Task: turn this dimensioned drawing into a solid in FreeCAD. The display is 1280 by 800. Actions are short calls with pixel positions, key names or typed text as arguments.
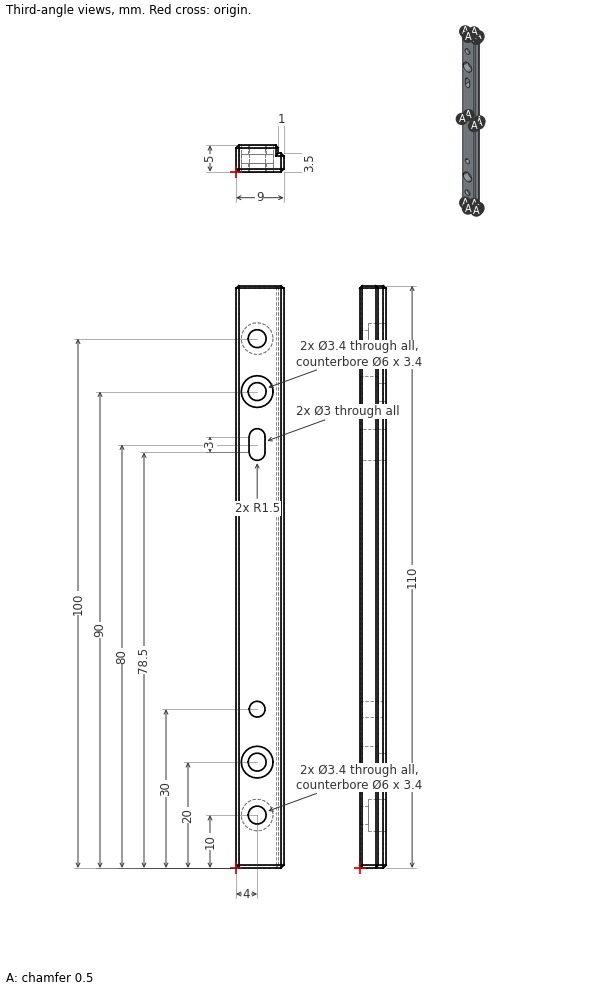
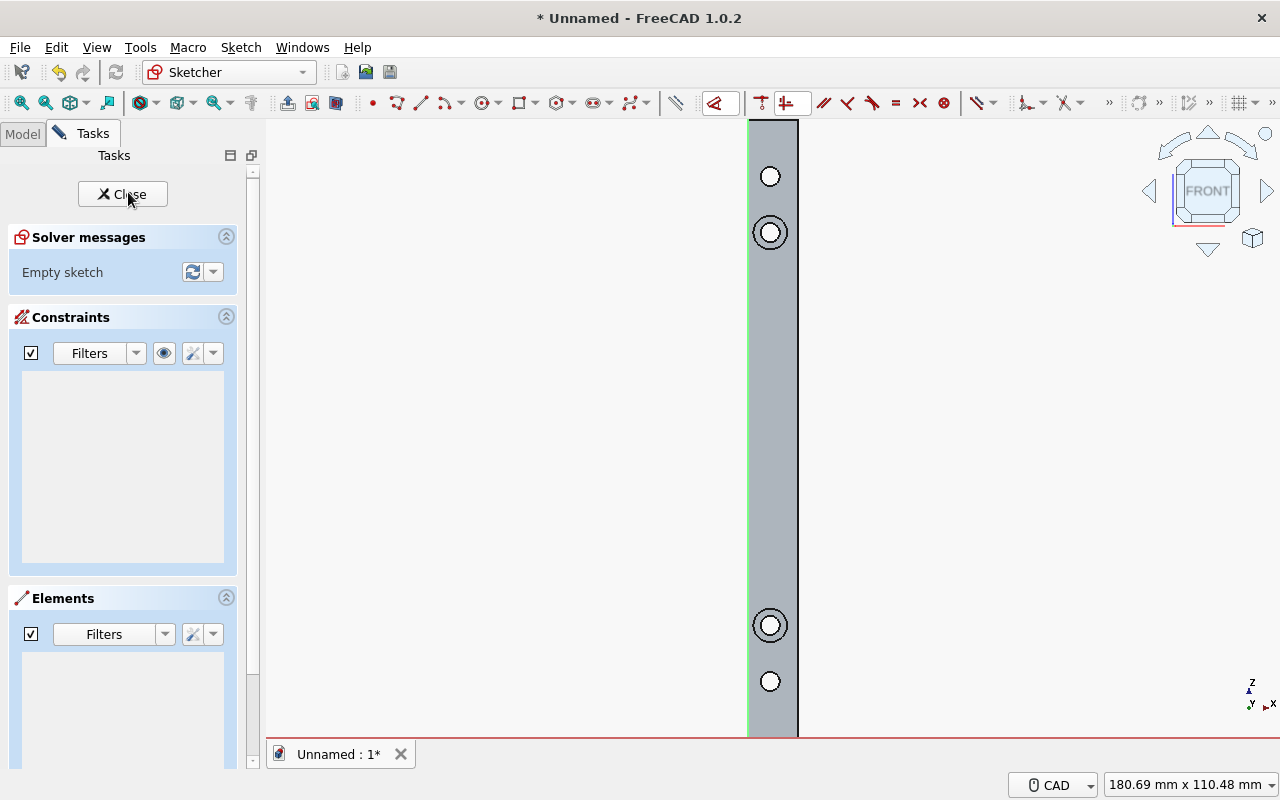
scroll(439, 147, down, 1)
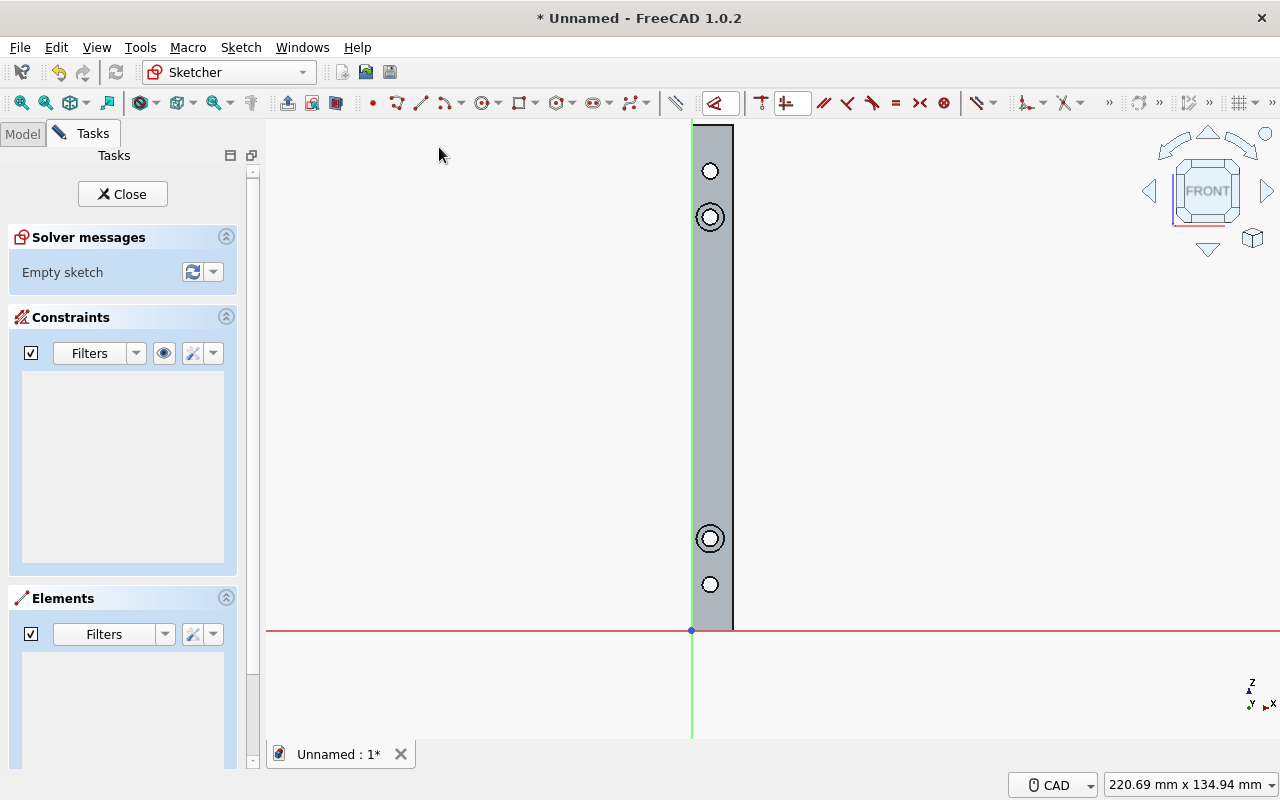
key(g)
key(c)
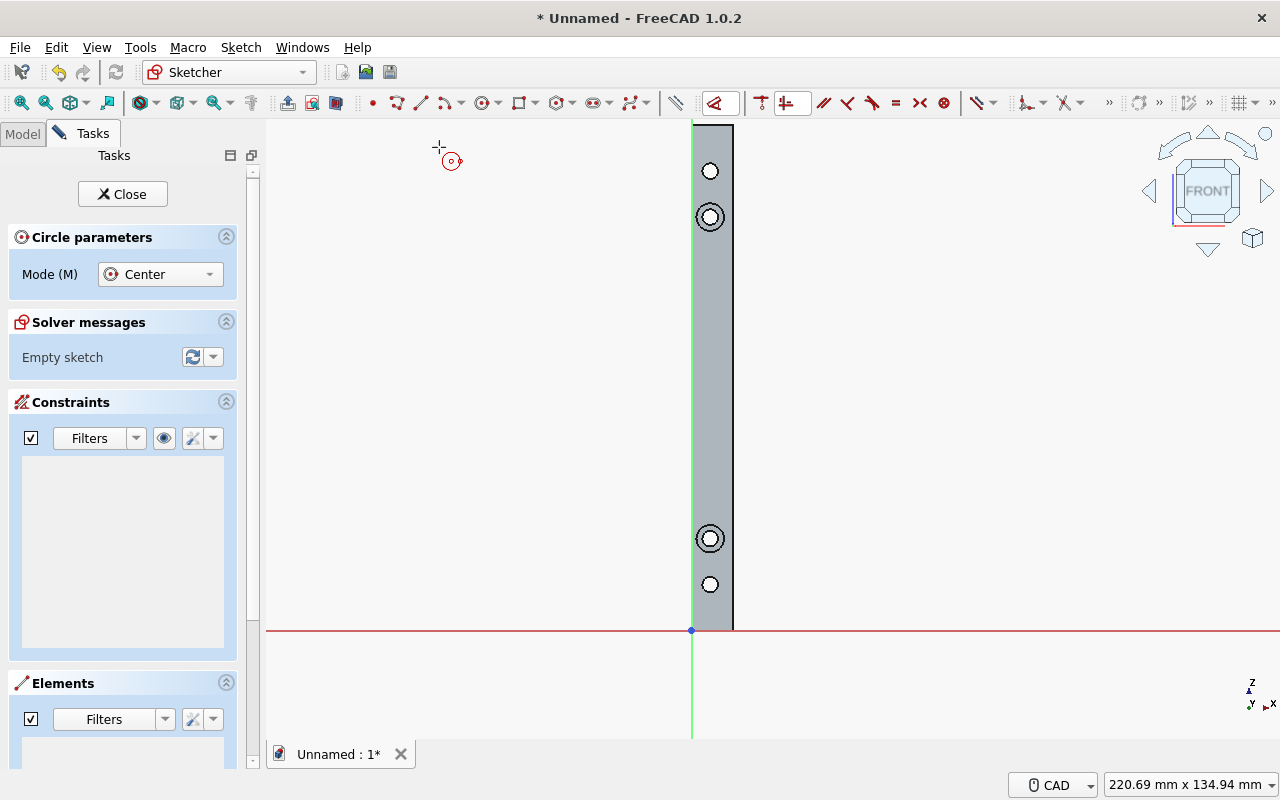
scroll(710, 263, up, 6)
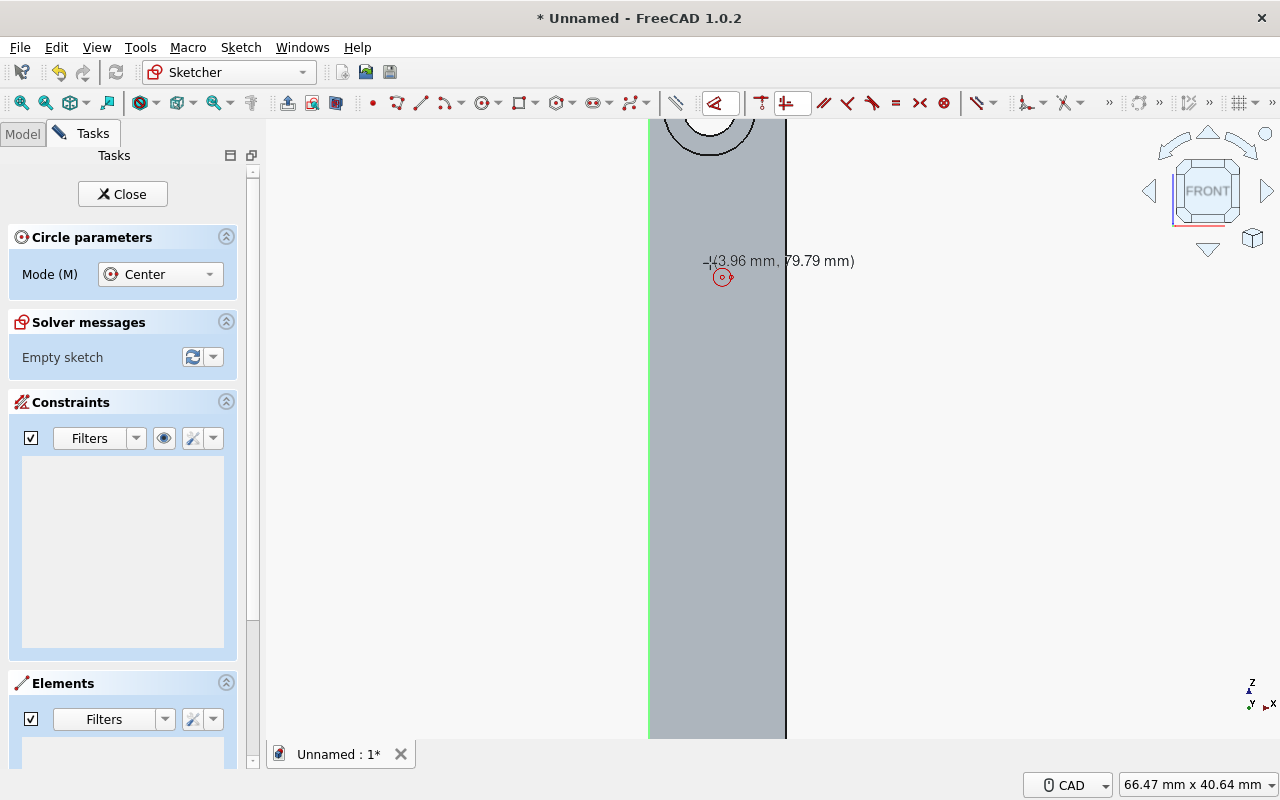
click(710, 263)
click(726, 246)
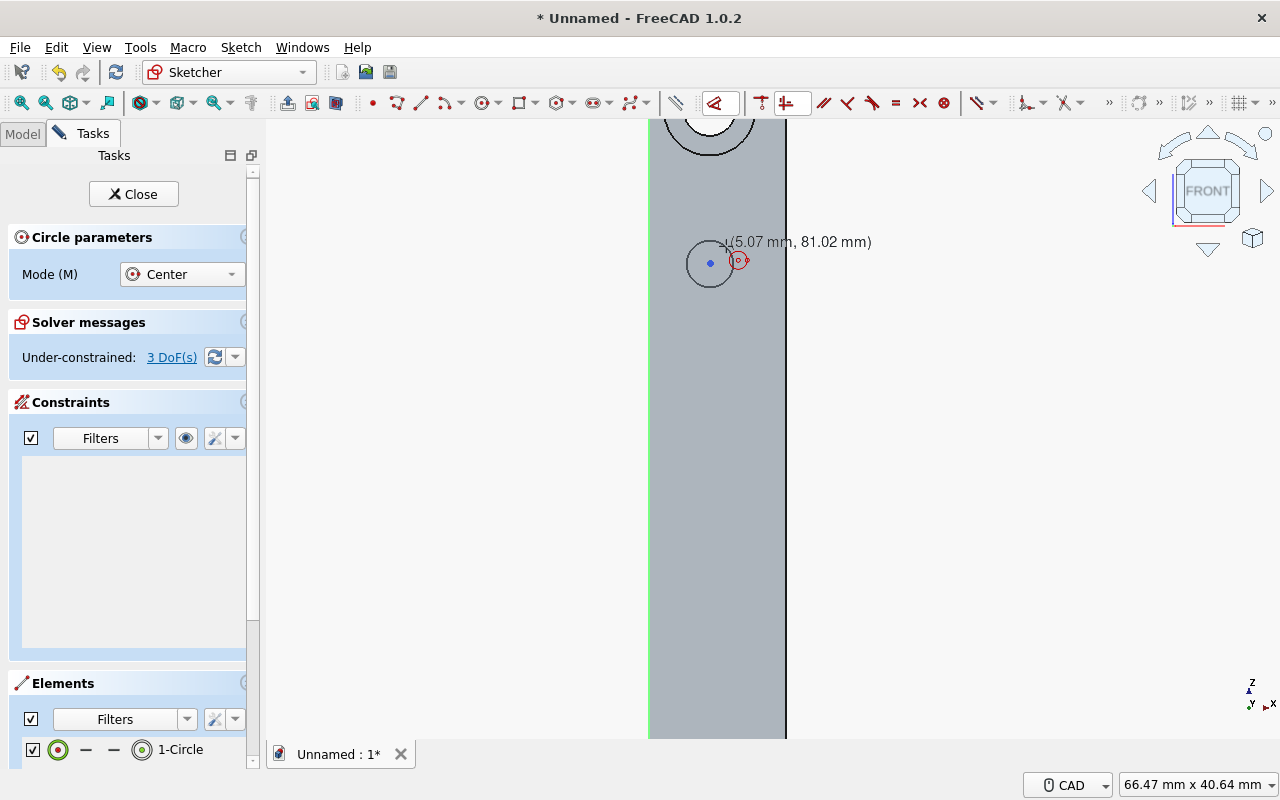
scroll(711, 243, down, 6)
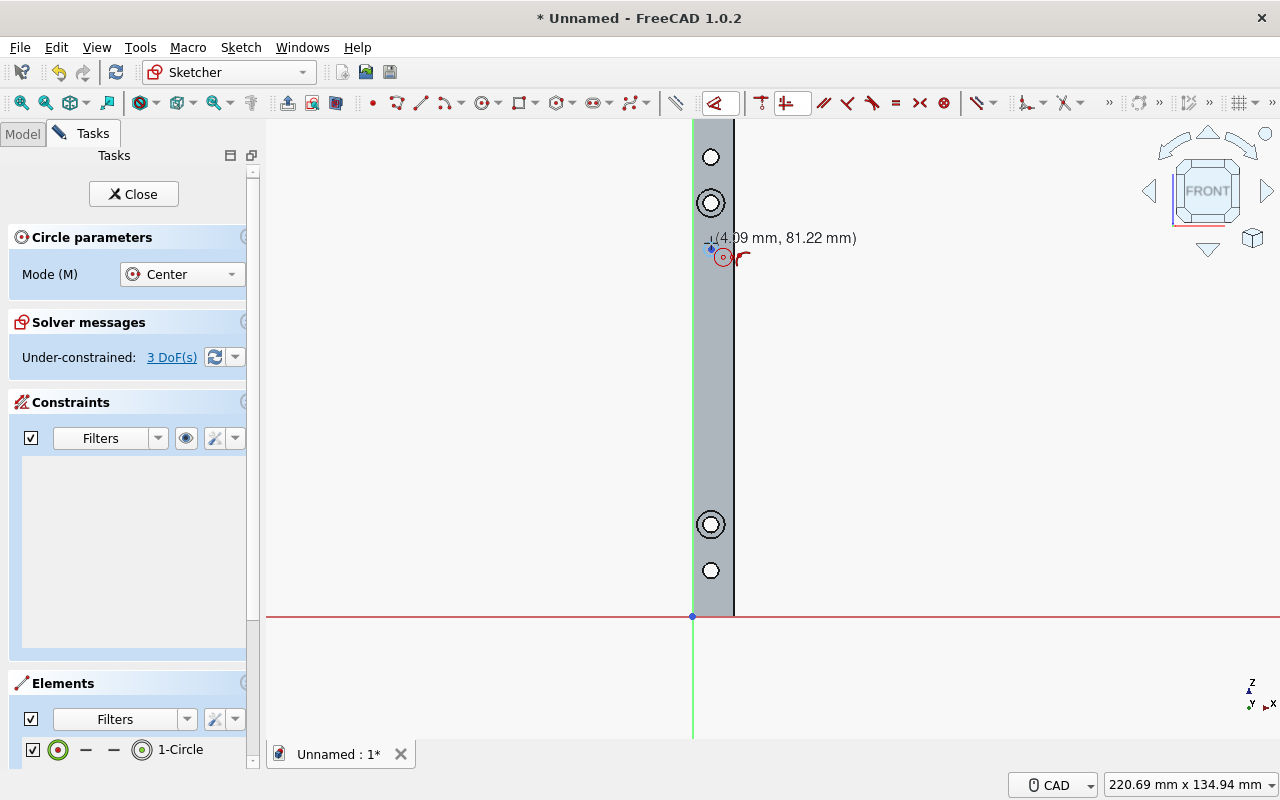
scroll(711, 479, up, 6)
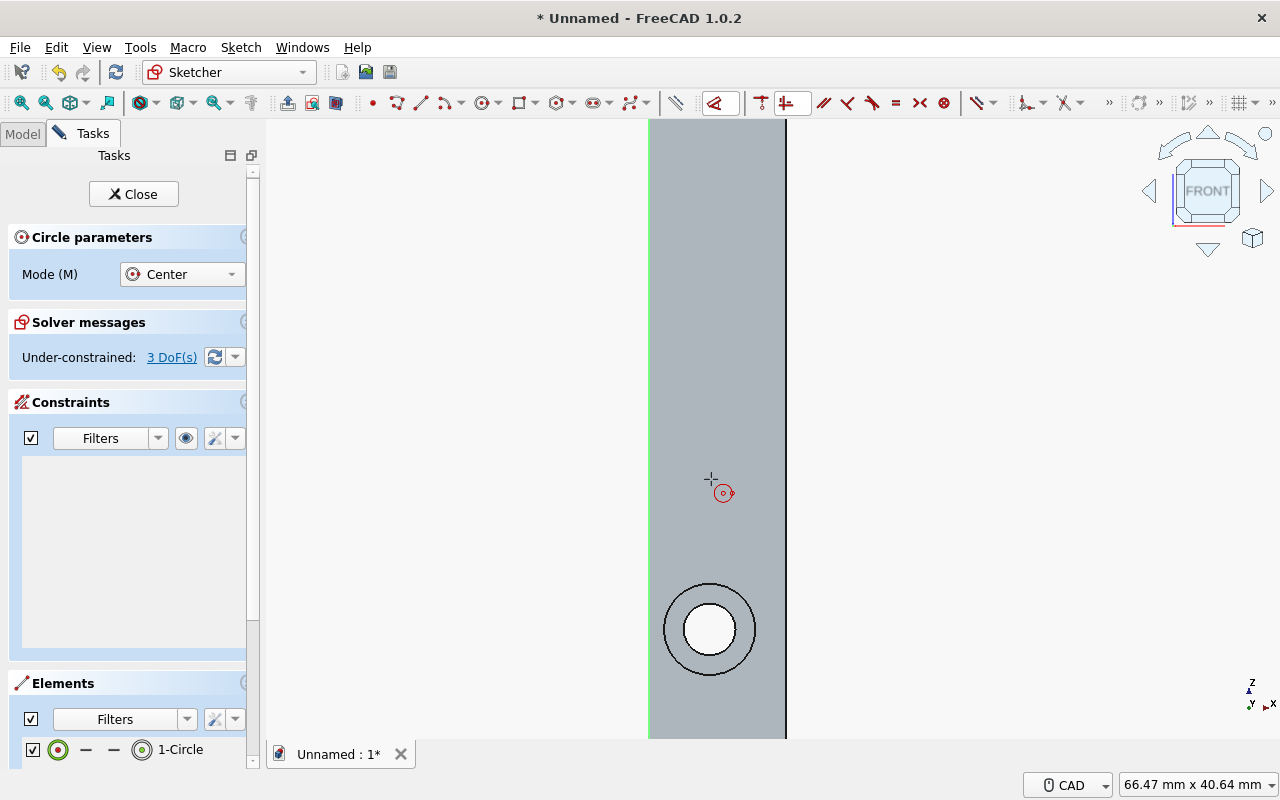
click(710, 477)
click(726, 461)
key(Escape)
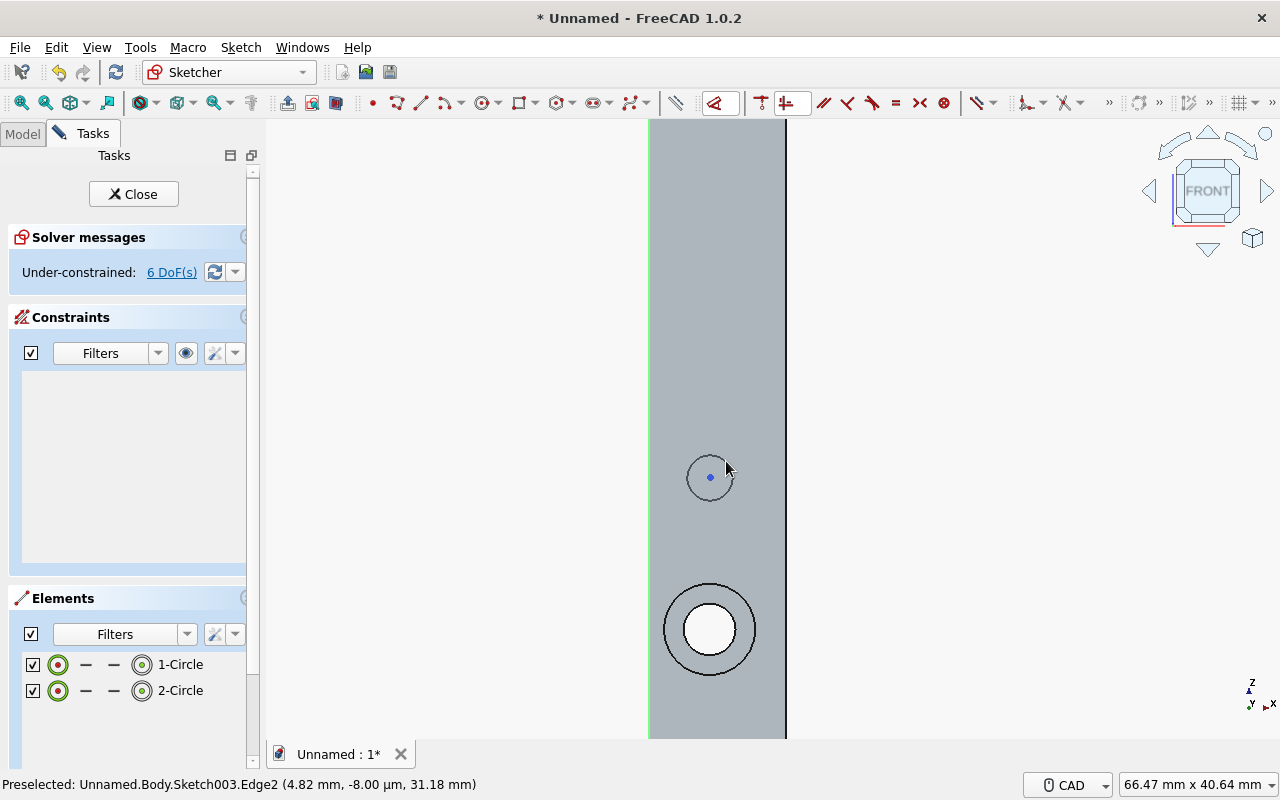
scroll(711, 479, down, 6)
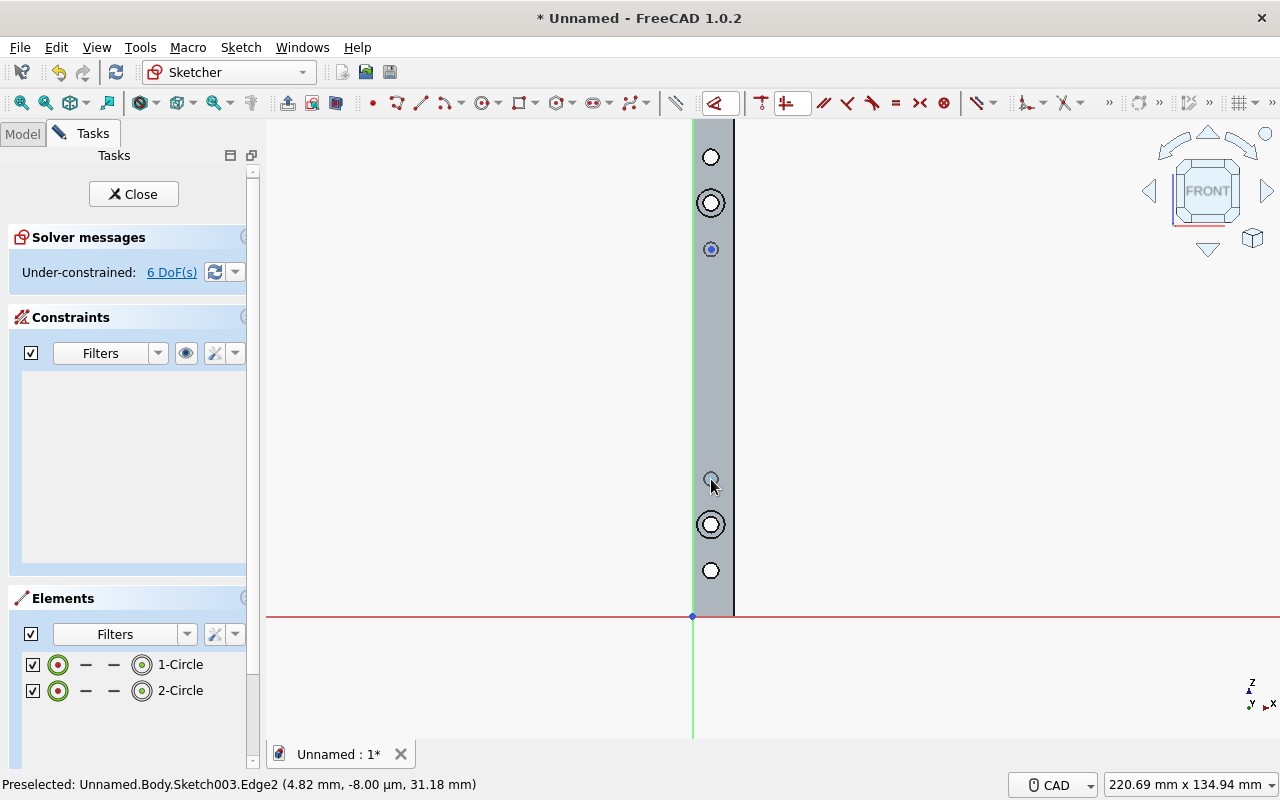
scroll(716, 244, up, 4)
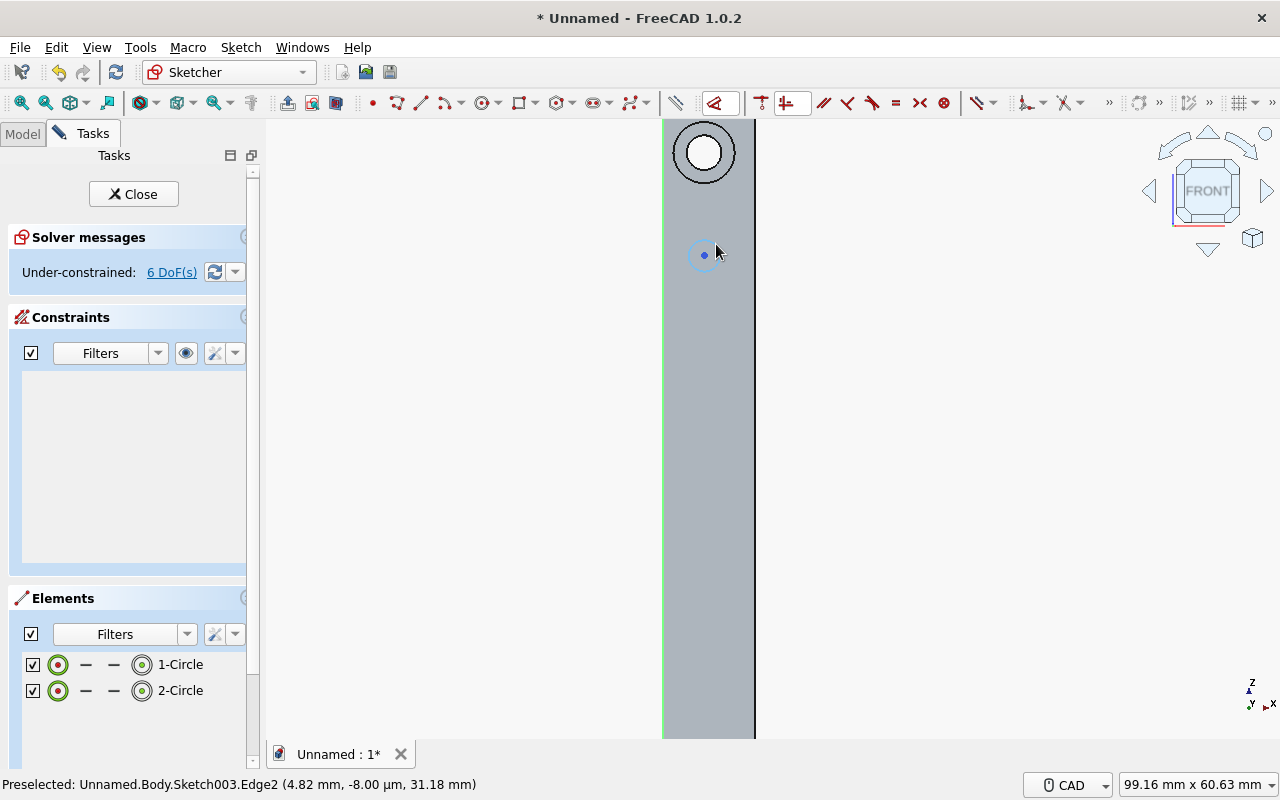
click(715, 245)